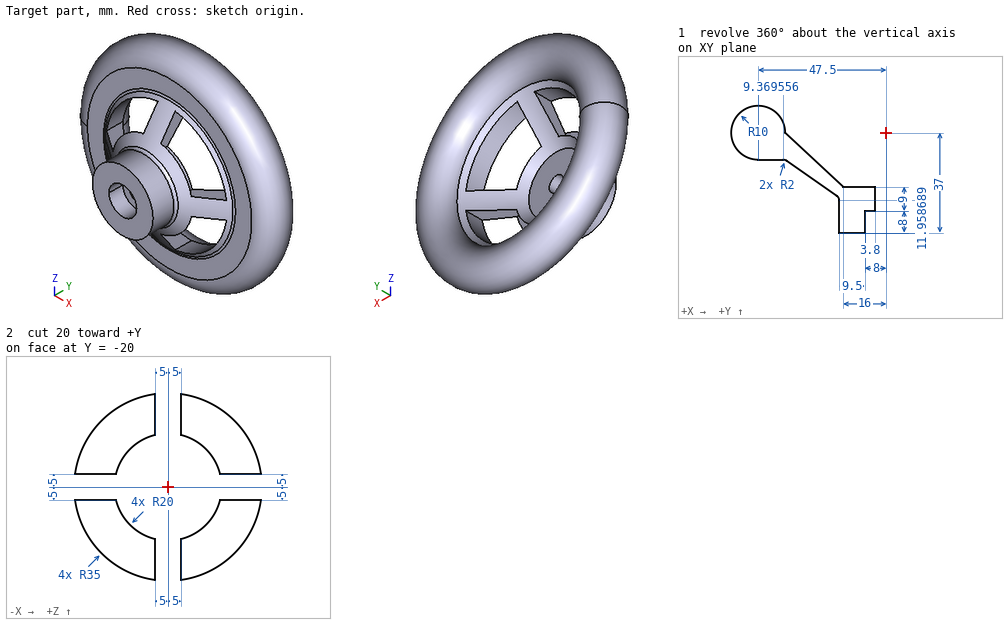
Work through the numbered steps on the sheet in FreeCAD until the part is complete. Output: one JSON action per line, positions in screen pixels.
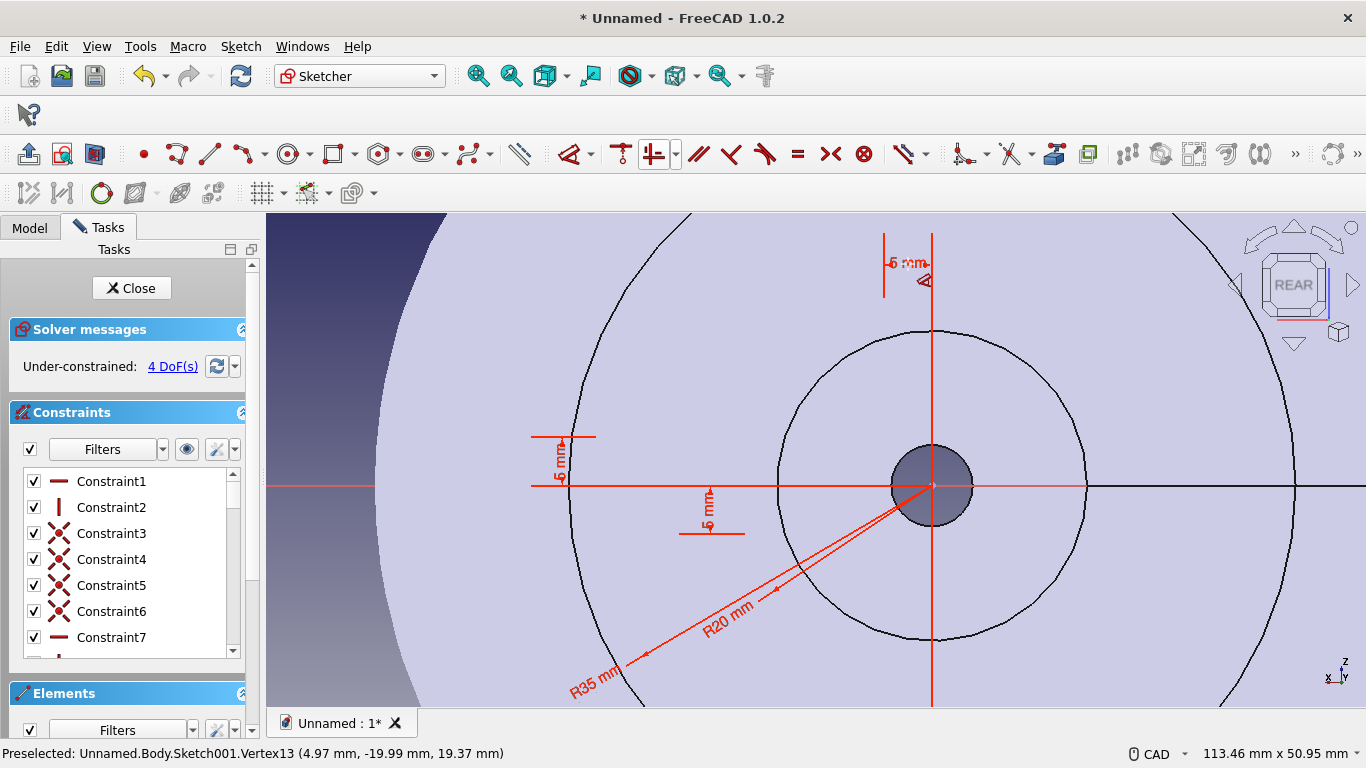
{"action": "scroll", "coordinate": [597, 439], "scroll_direction": "down", "scroll_amount": 4}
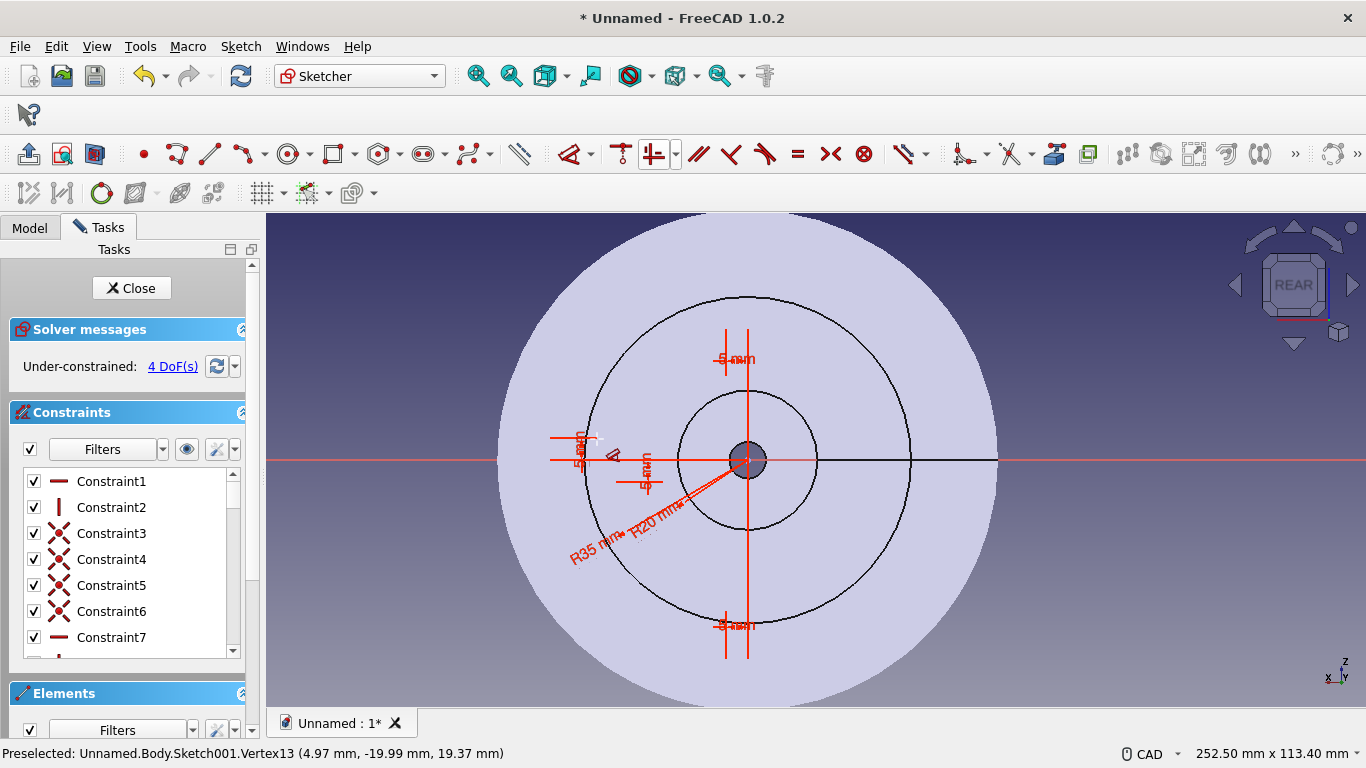
{"action": "scroll", "coordinate": [899, 483], "scroll_direction": "up", "scroll_amount": 4}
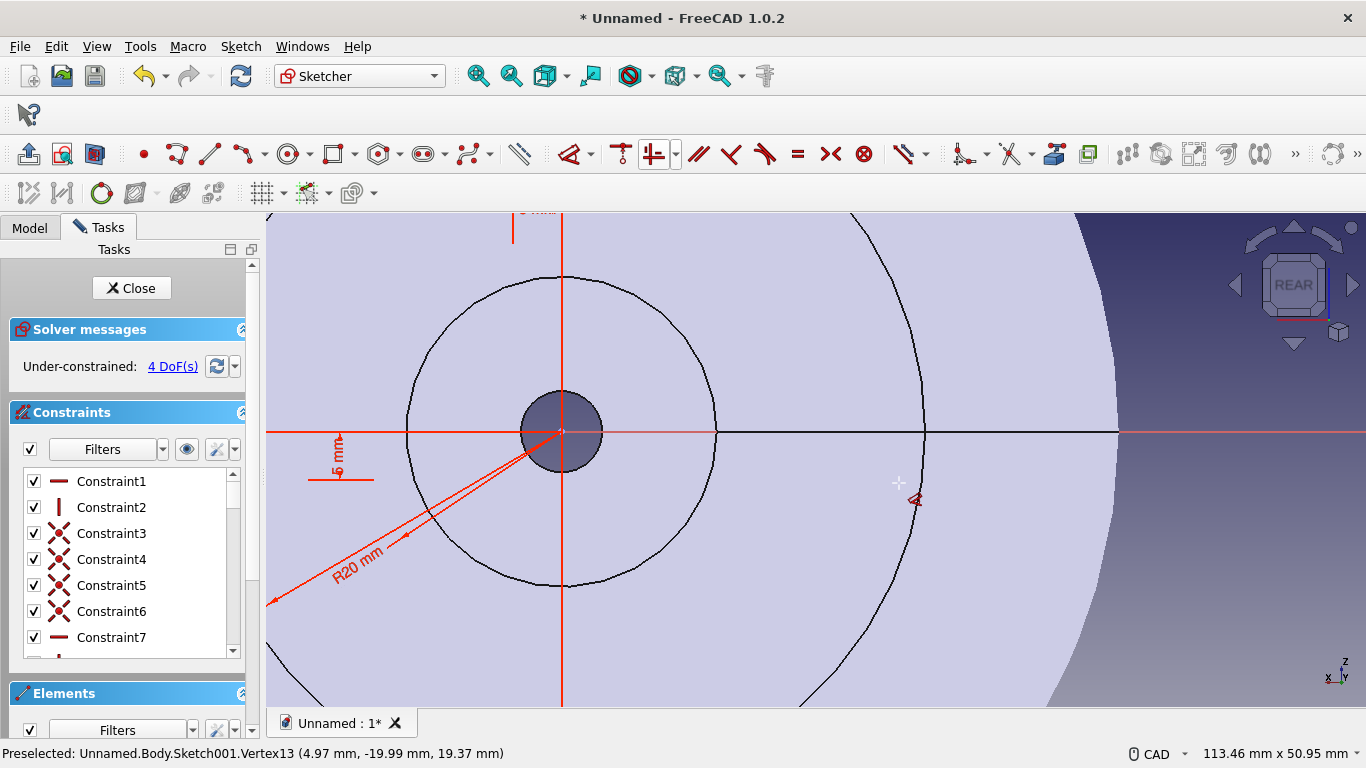
{"action": "left_click", "coordinate": [897, 482]}
{"action": "left_click", "coordinate": [931, 457]}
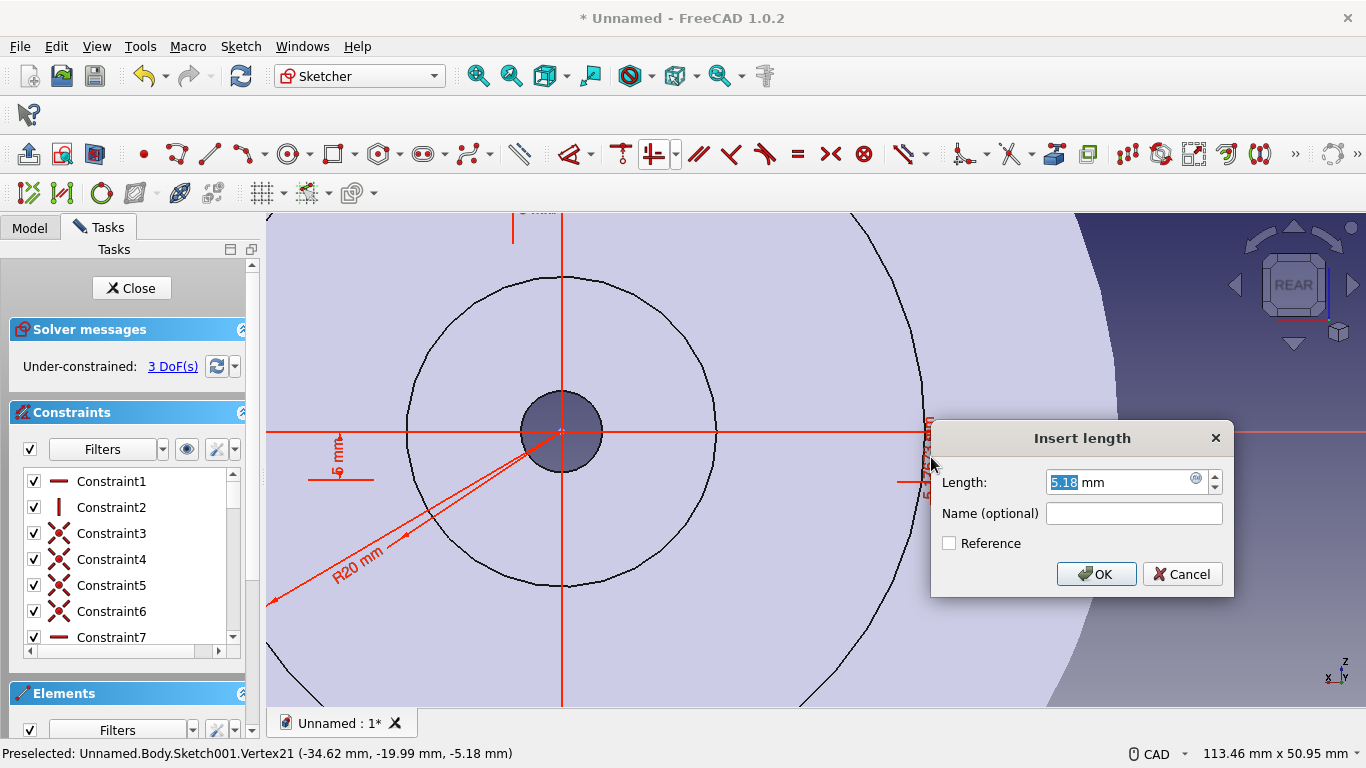
{"action": "type", "text": "5"}
{"action": "key", "text": "Return"}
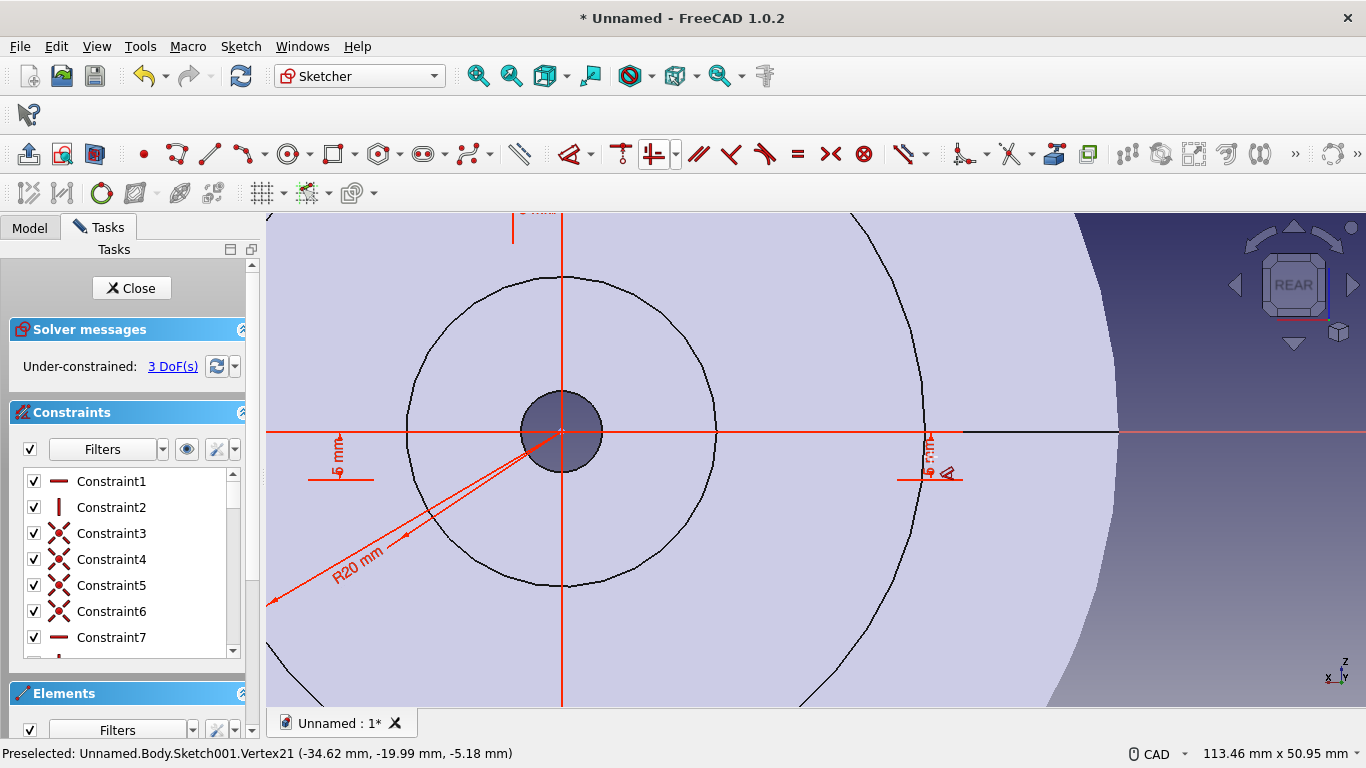
{"action": "left_click", "coordinate": [610, 620]}
{"action": "left_click", "coordinate": [586, 654]}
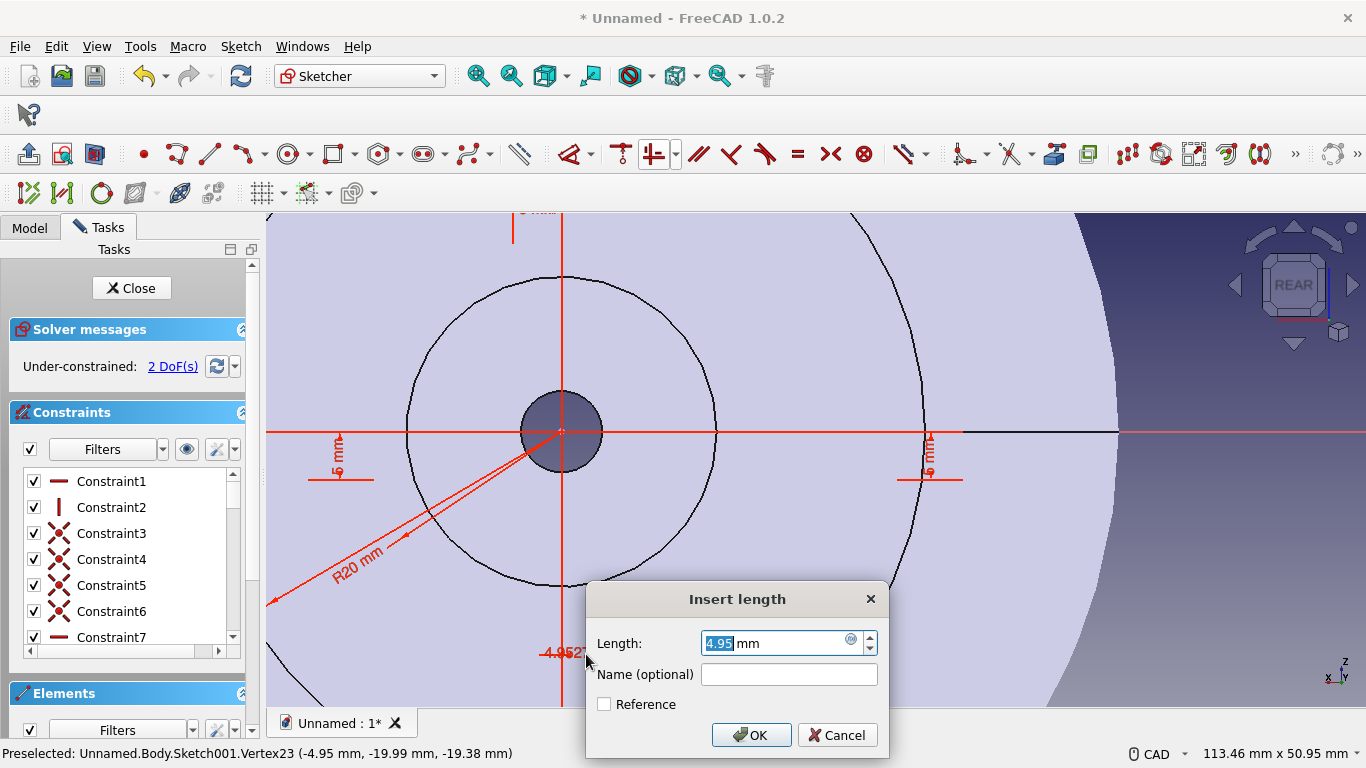
{"action": "type", "text": "5"}
{"action": "key", "text": "Return"}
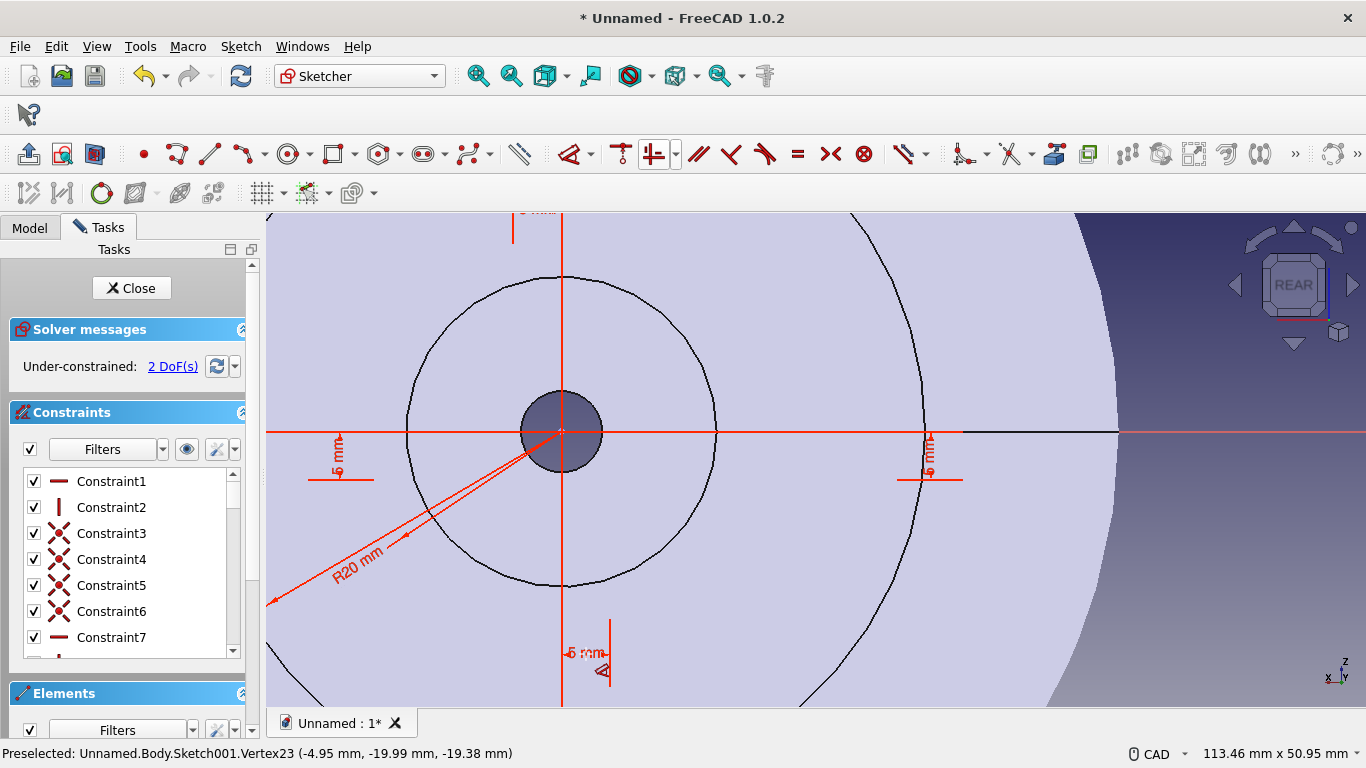
{"action": "scroll", "coordinate": [899, 483], "scroll_direction": "down", "scroll_amount": 4}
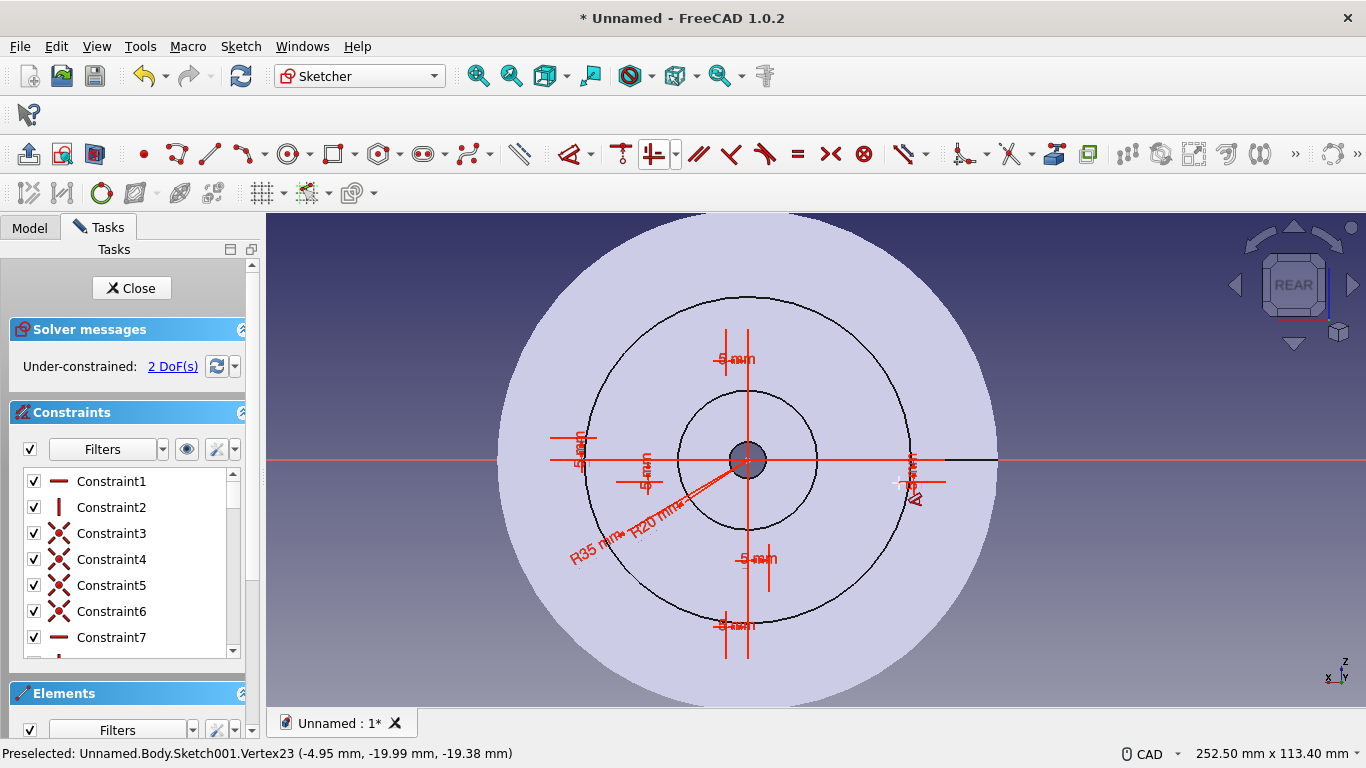
{"action": "scroll", "coordinate": [769, 309], "scroll_direction": "up", "scroll_amount": 4}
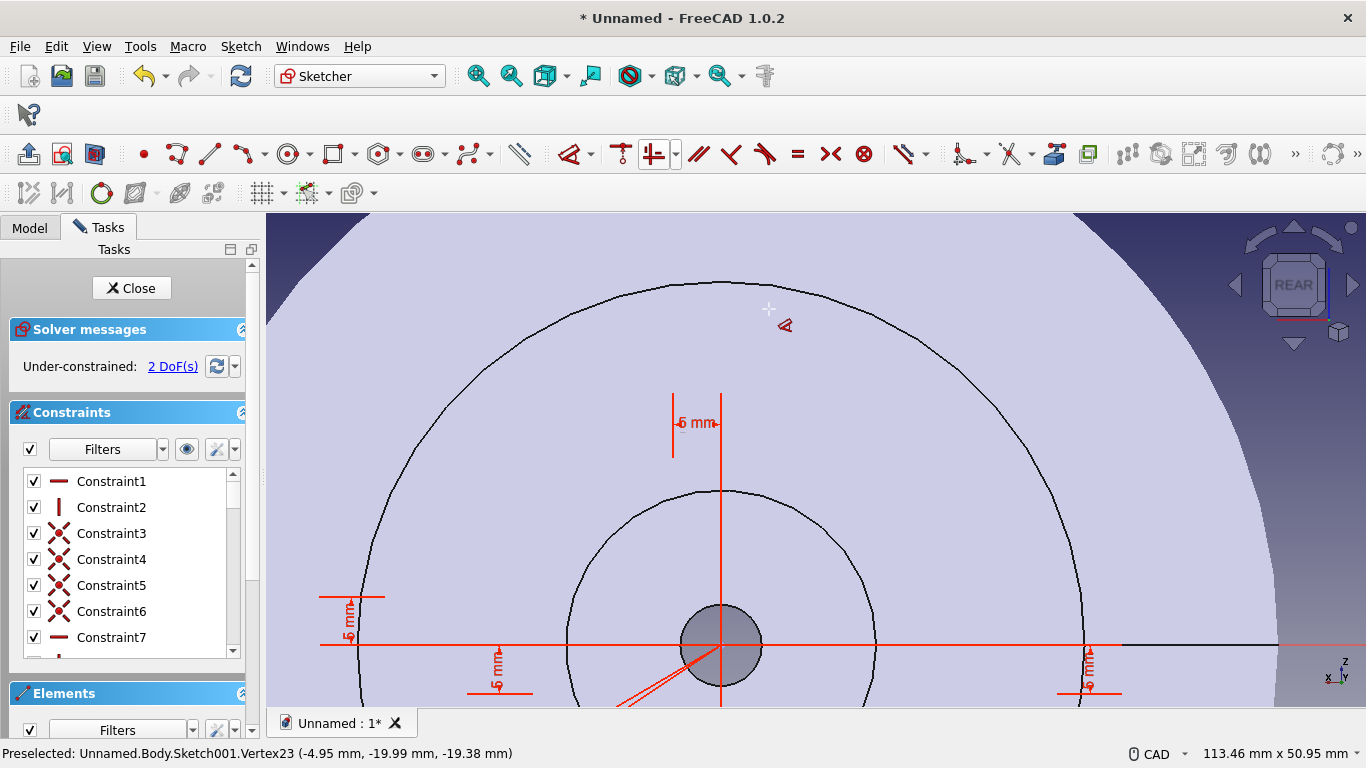
{"action": "left_click", "coordinate": [769, 309]}
{"action": "left_click", "coordinate": [745, 275]}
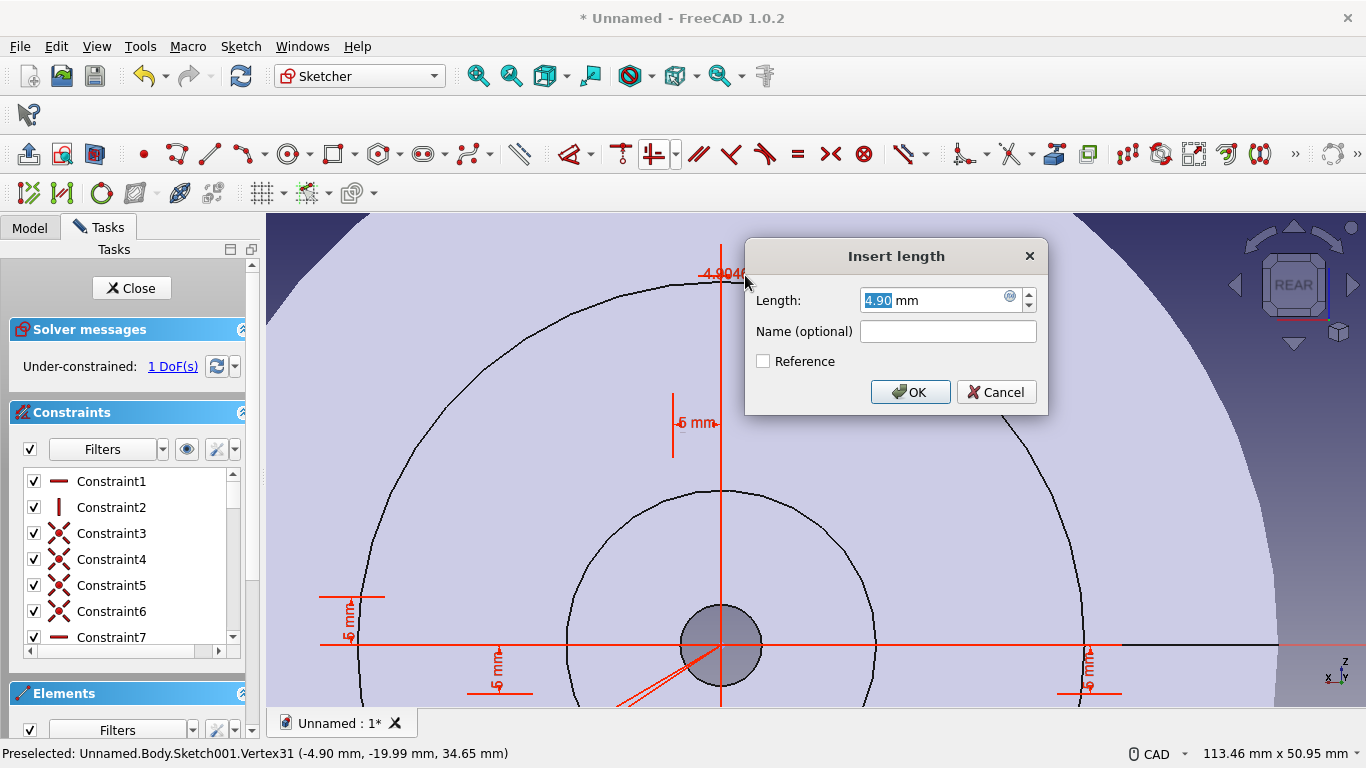
{"action": "type", "text": "5"}
{"action": "key", "text": "Return"}